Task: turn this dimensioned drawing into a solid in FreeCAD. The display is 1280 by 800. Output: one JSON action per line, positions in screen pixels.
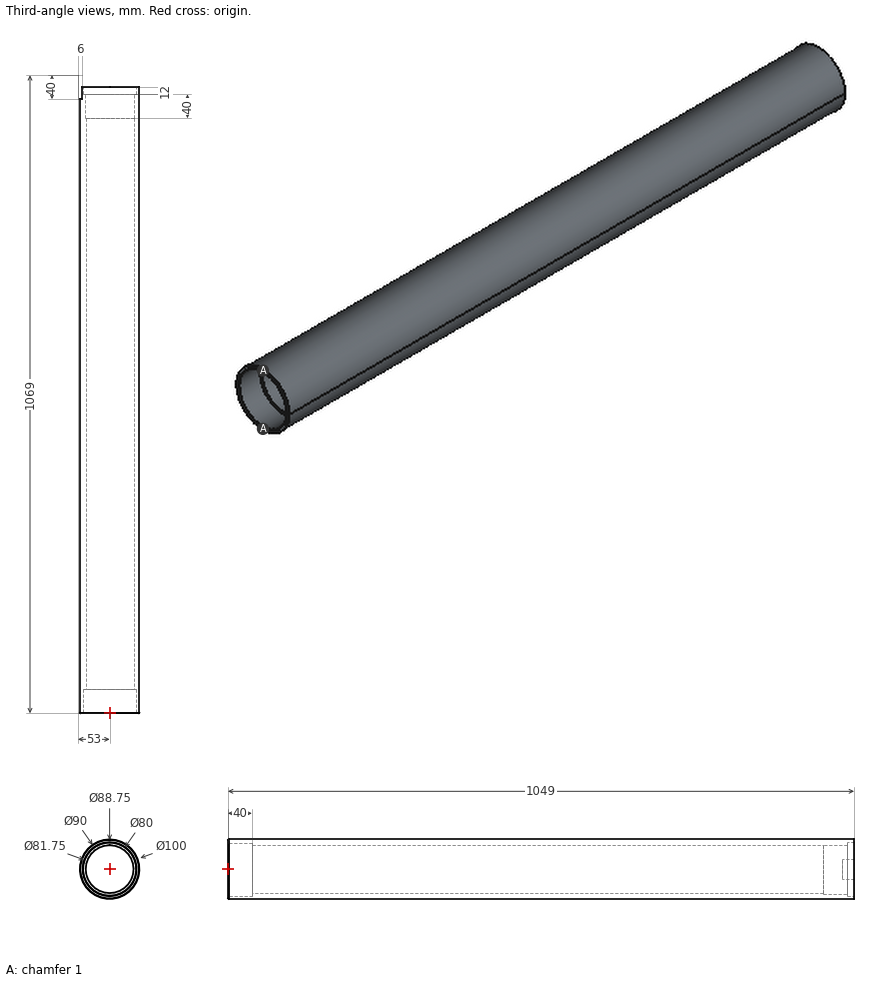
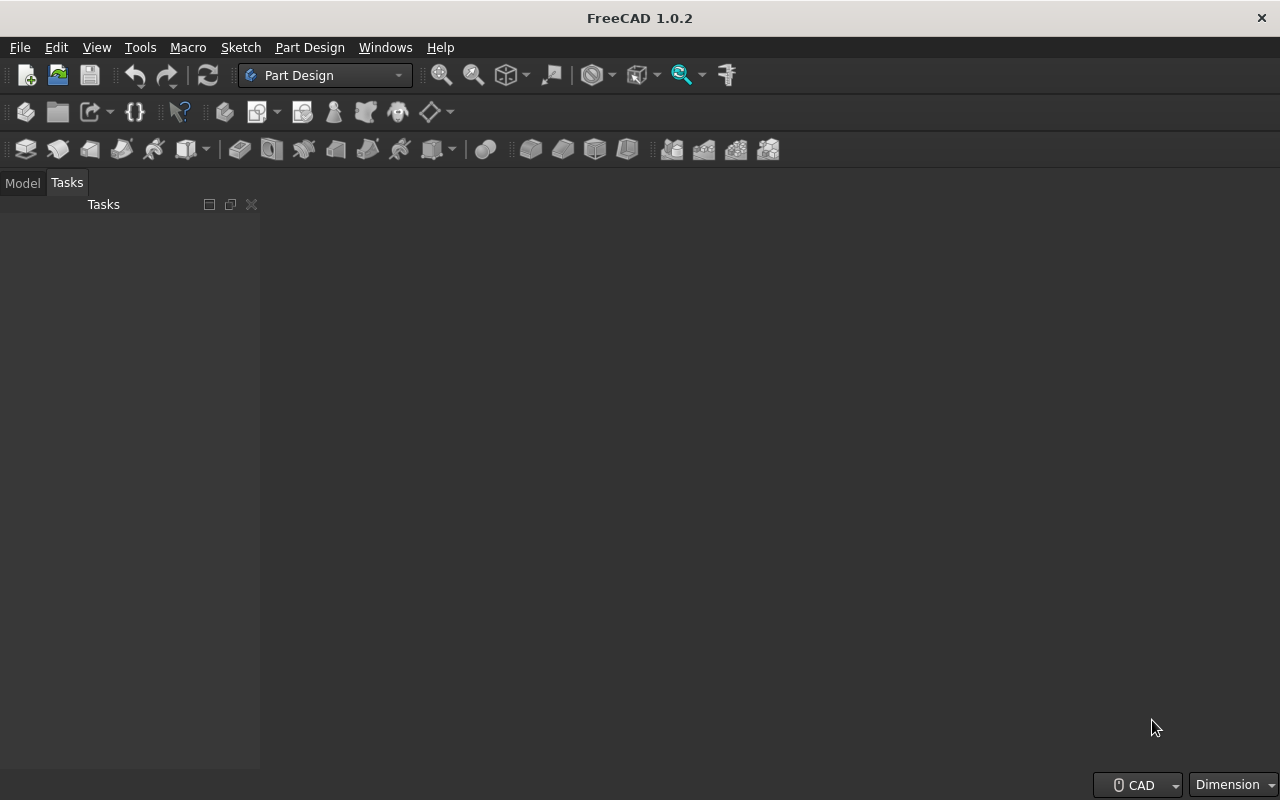
{"action": "left_click", "coordinate": [26, 76]}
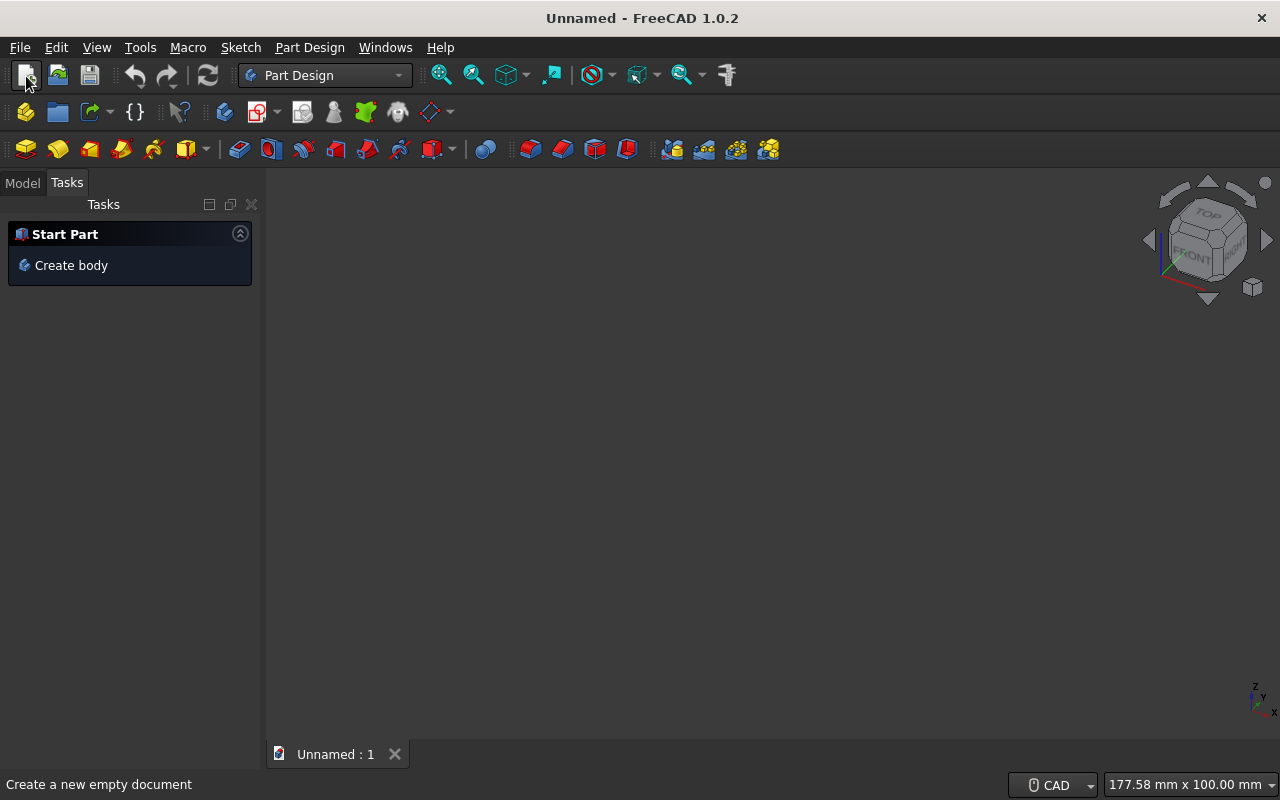
{"action": "left_click", "coordinate": [258, 112]}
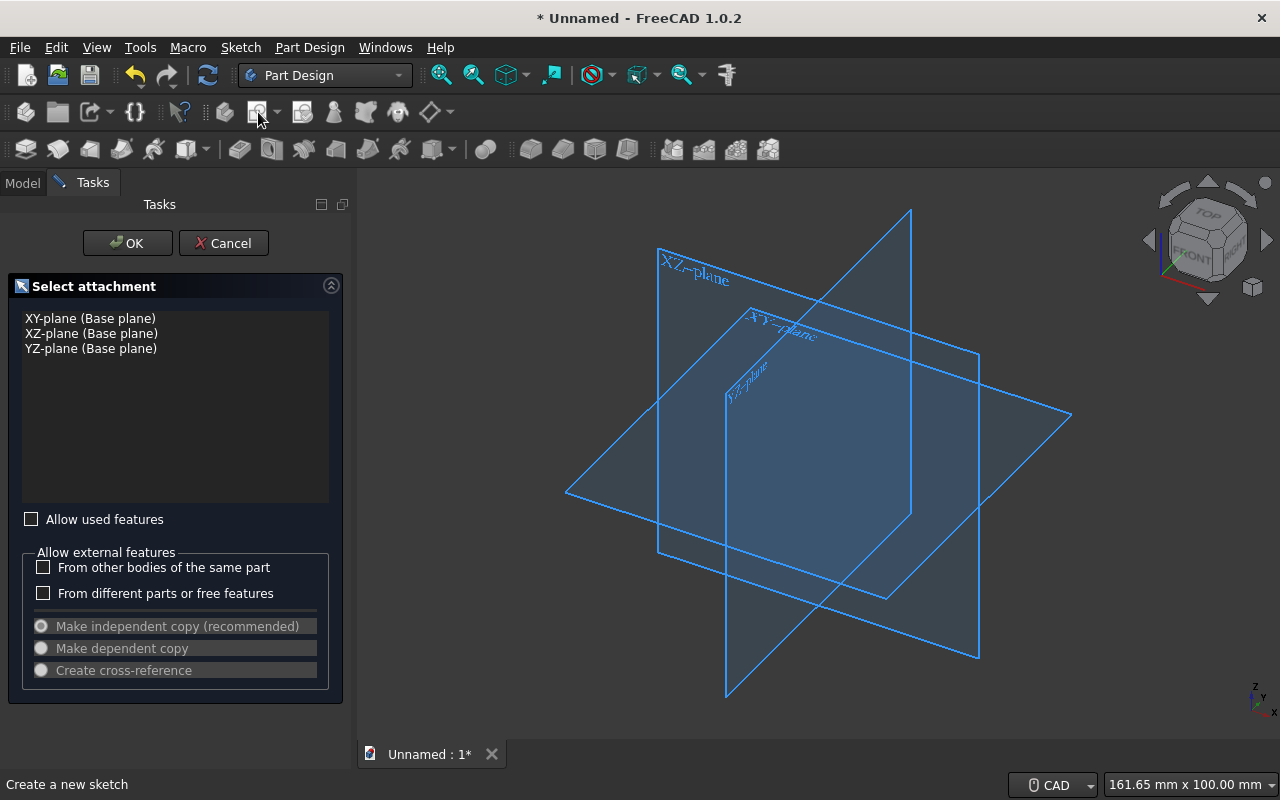
{"action": "left_click", "coordinate": [82, 334]}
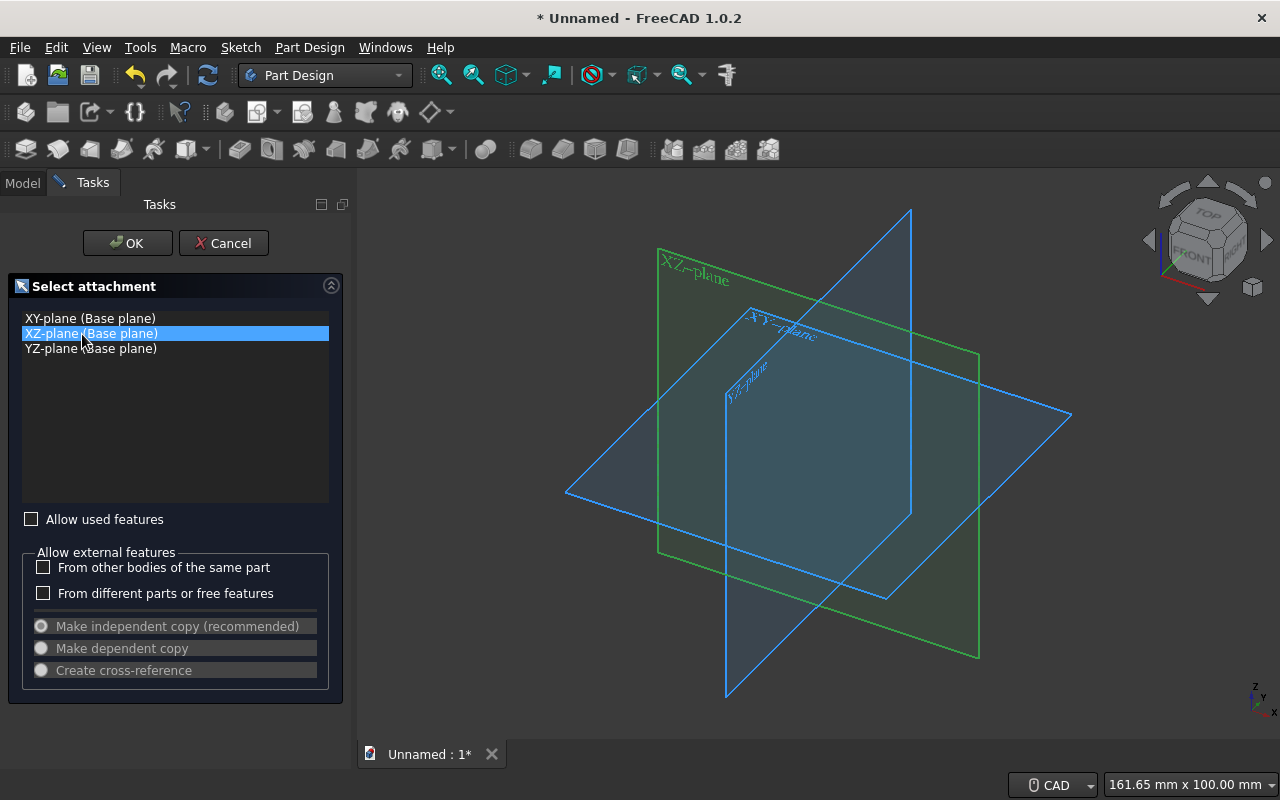
{"action": "left_click", "coordinate": [128, 243]}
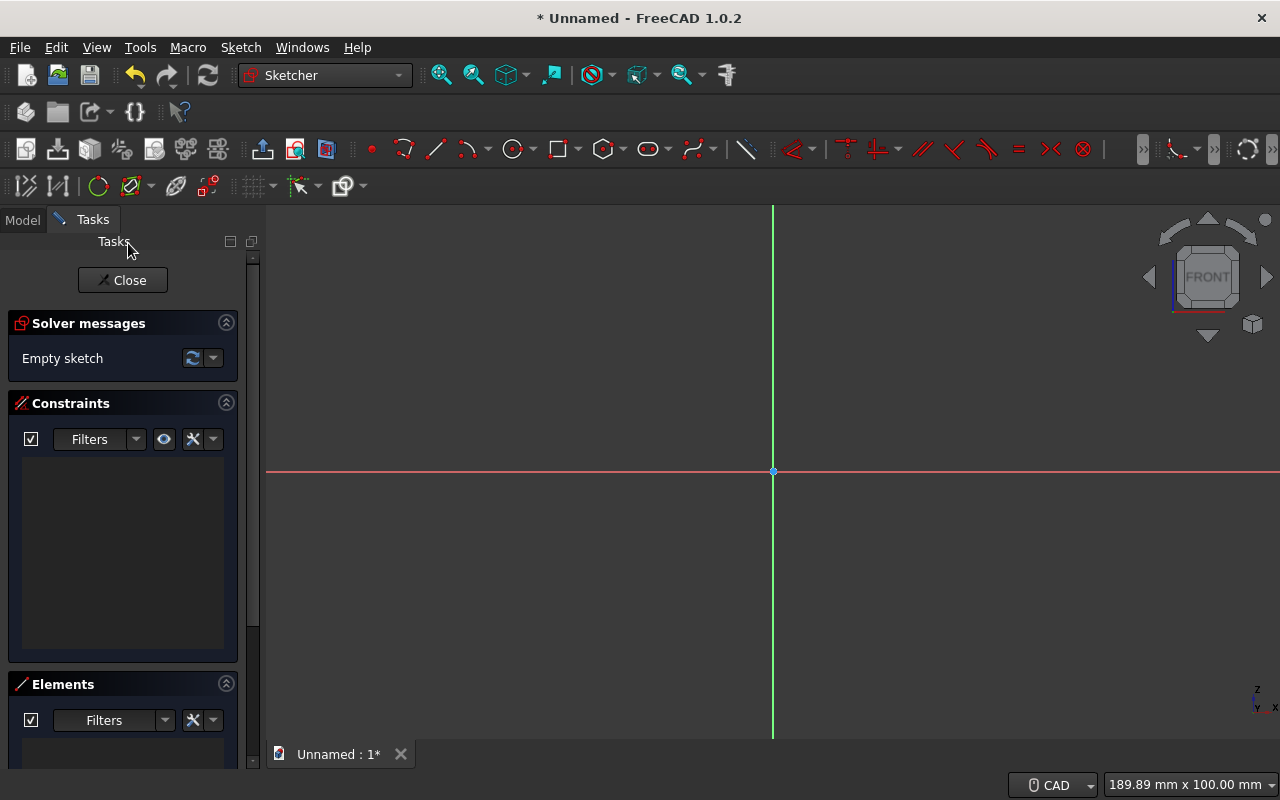
{"action": "scroll", "coordinate": [565, 472], "scroll_direction": "down", "scroll_amount": 2}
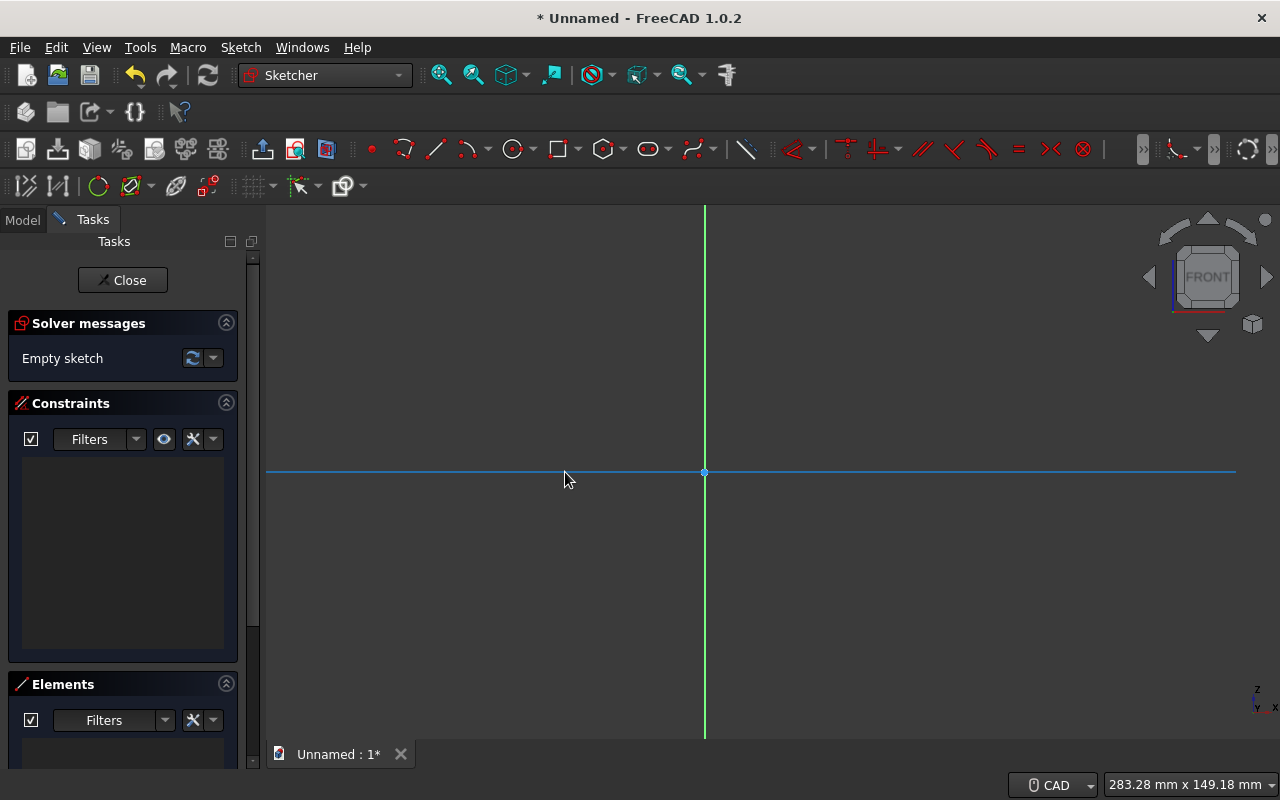
{"action": "left_click", "coordinate": [514, 150]}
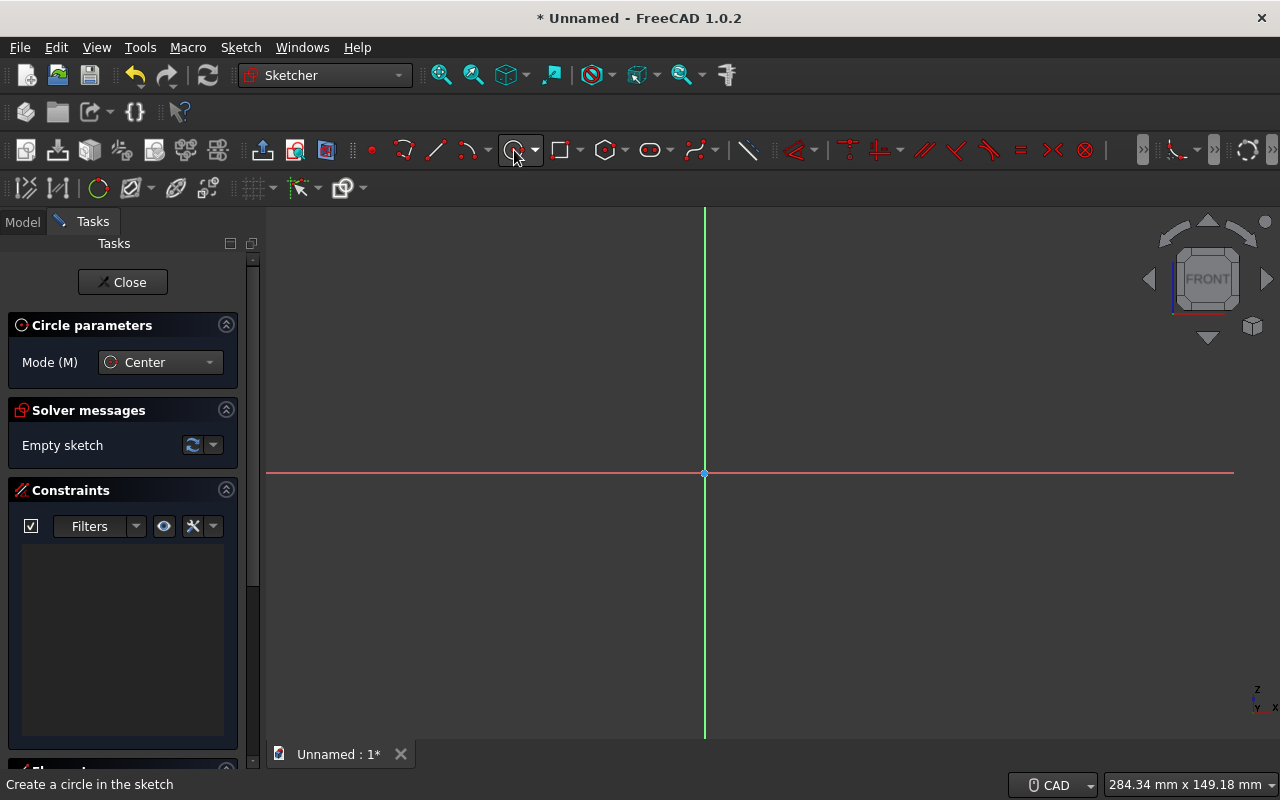
{"action": "left_click", "coordinate": [705, 473]}
{"action": "mouse_move", "coordinate": [831, 347]}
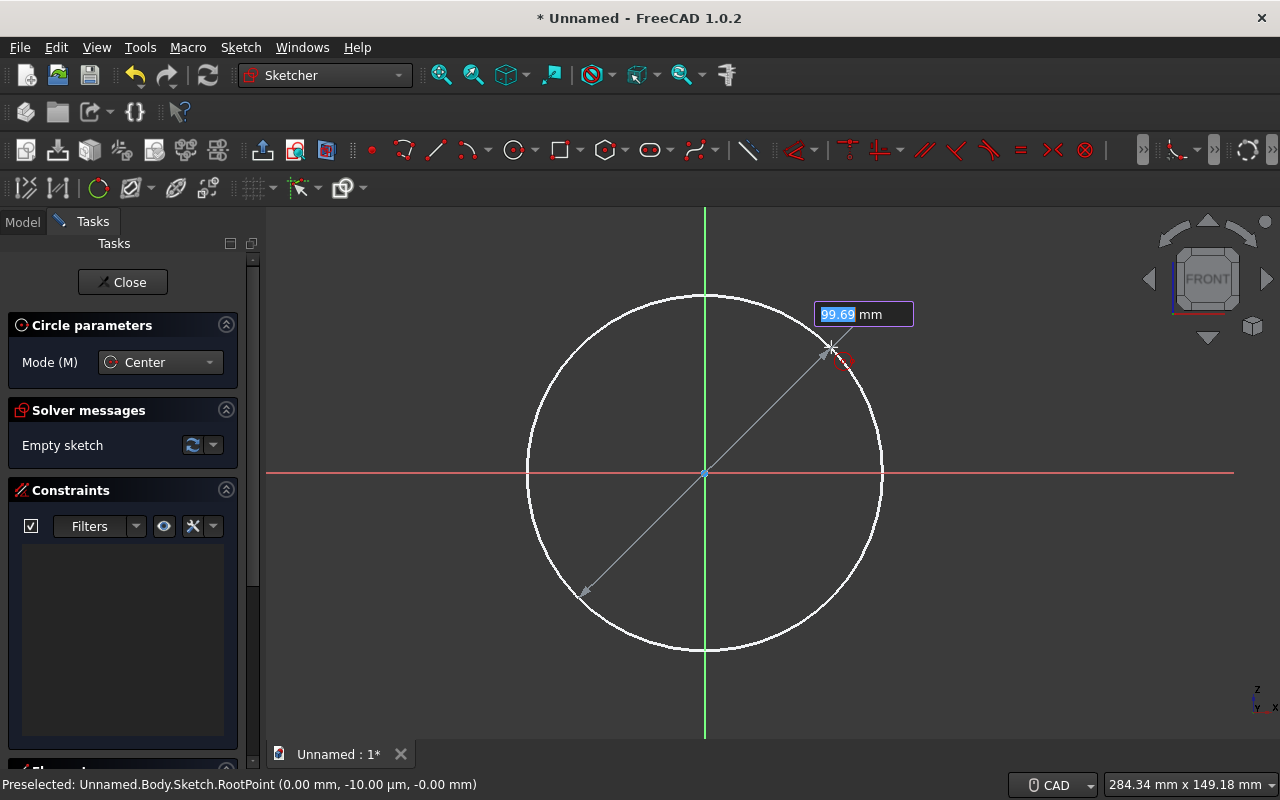
{"action": "type", "text": "100"}
{"action": "key", "text": "Return"}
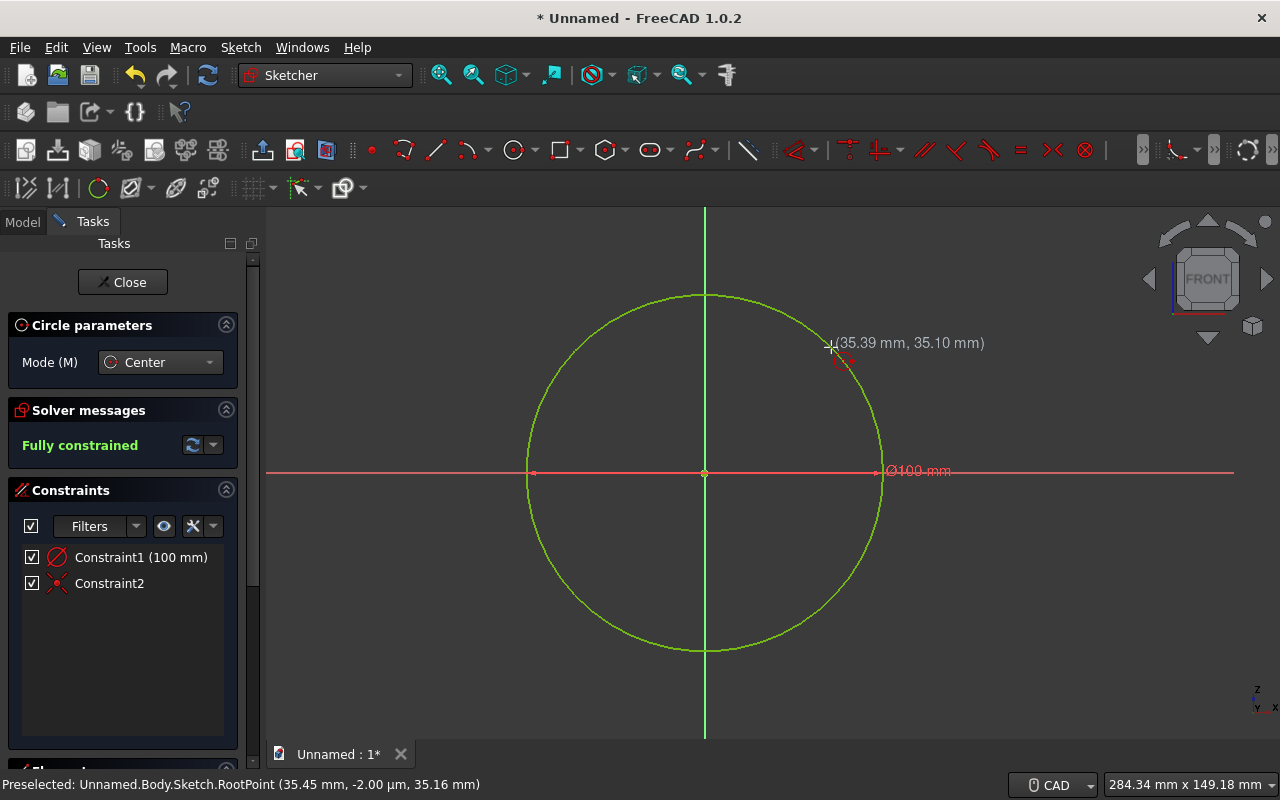
{"action": "left_click", "coordinate": [705, 473]}
{"action": "mouse_move", "coordinate": [806, 372]}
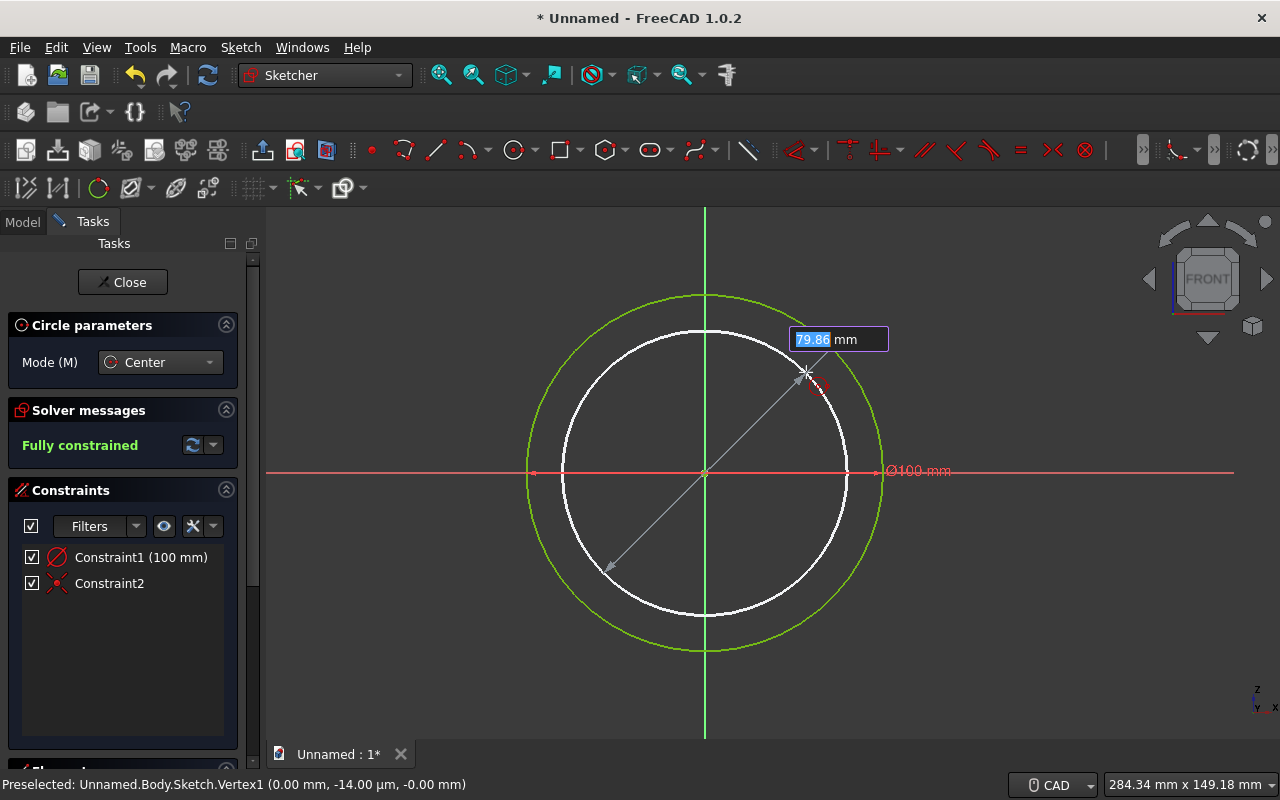
{"action": "type", "text": "80"}
{"action": "key", "text": "Return"}
{"action": "key", "text": "Escape"}